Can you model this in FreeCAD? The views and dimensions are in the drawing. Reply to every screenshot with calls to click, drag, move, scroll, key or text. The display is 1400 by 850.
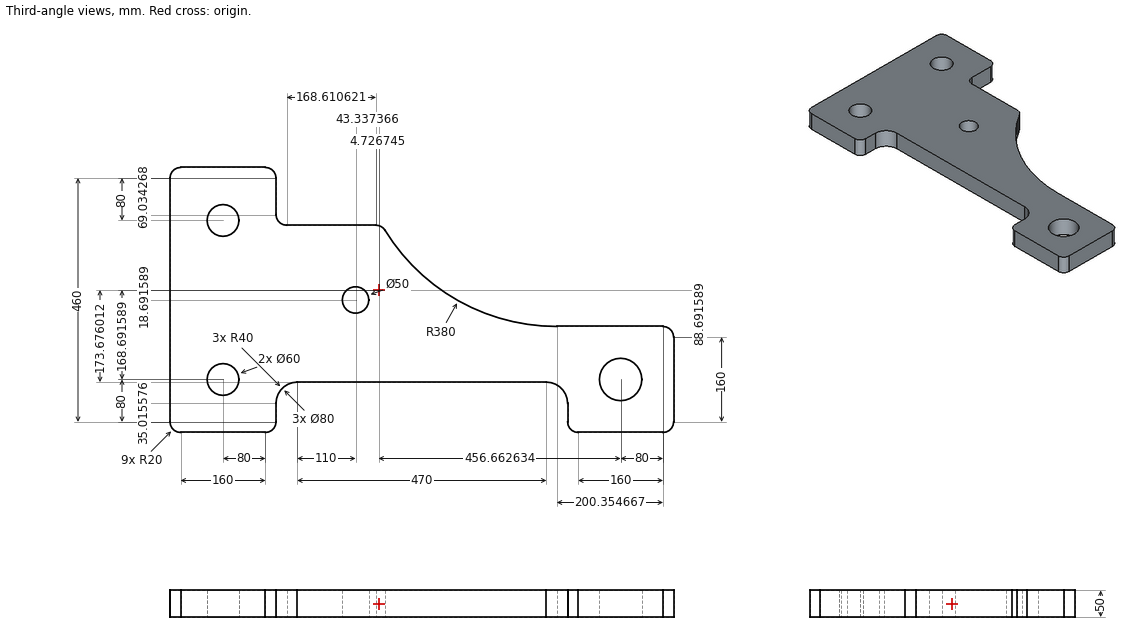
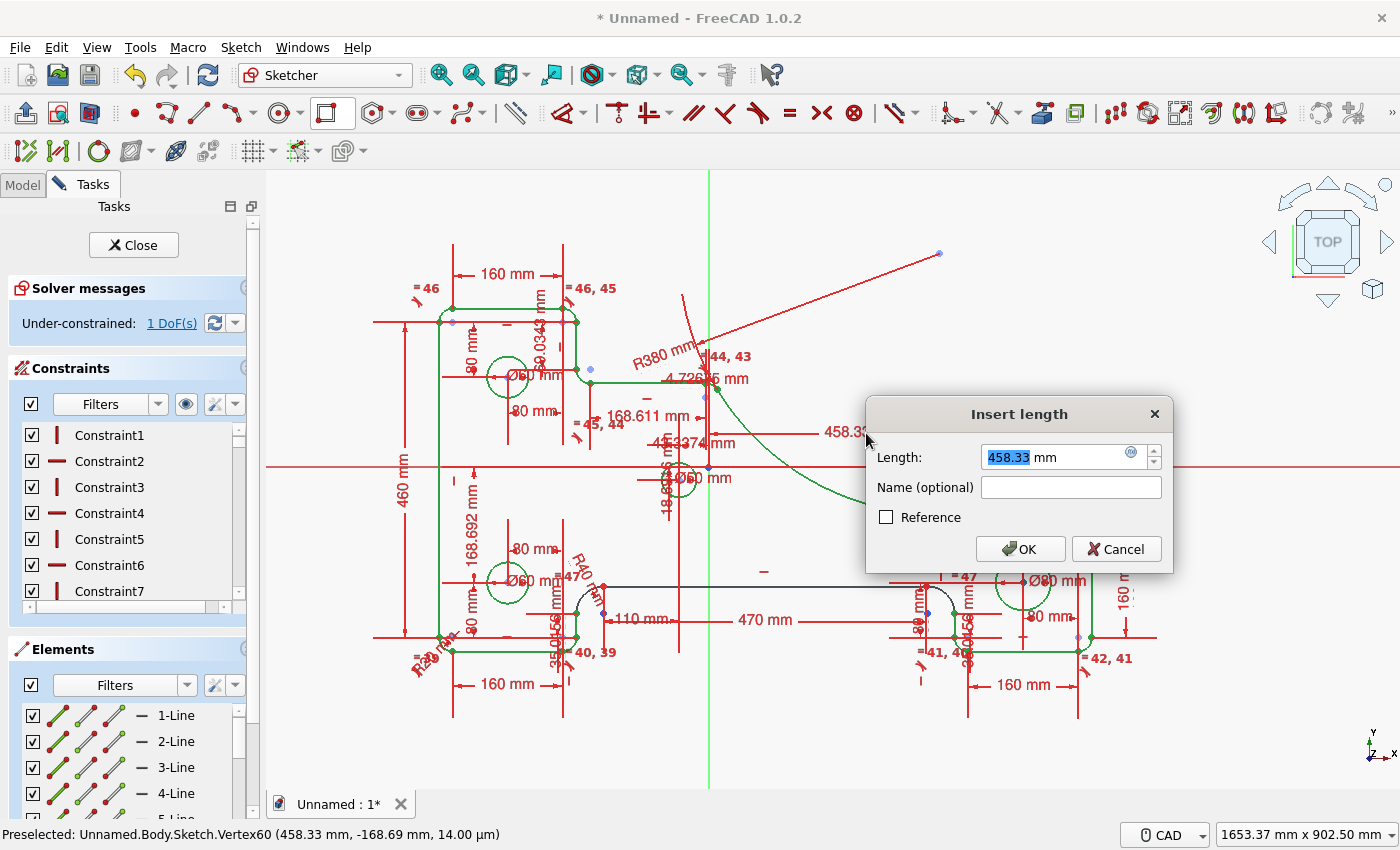
text(456.662634)
key(Return)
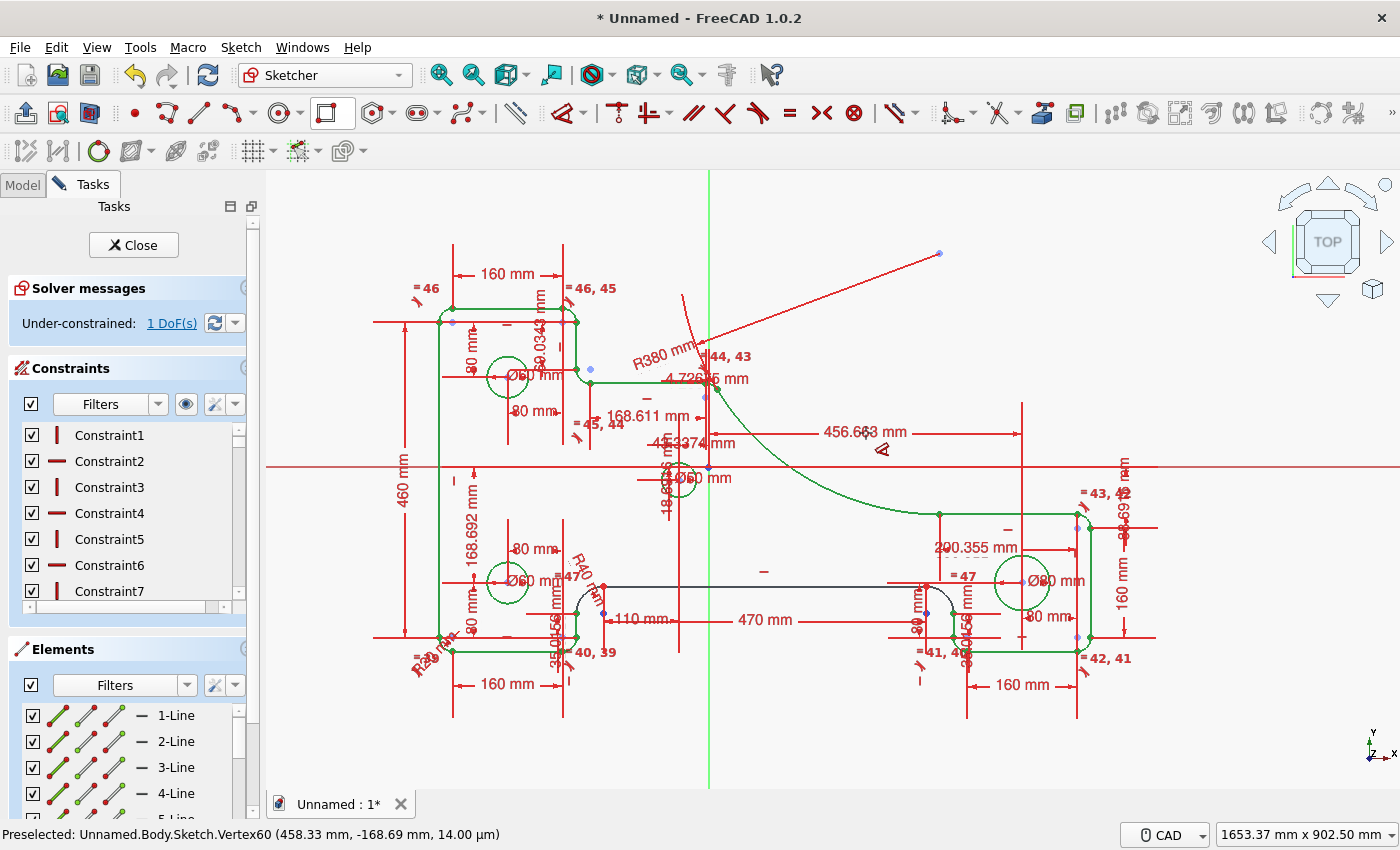
click(604, 587)
click(570, 527)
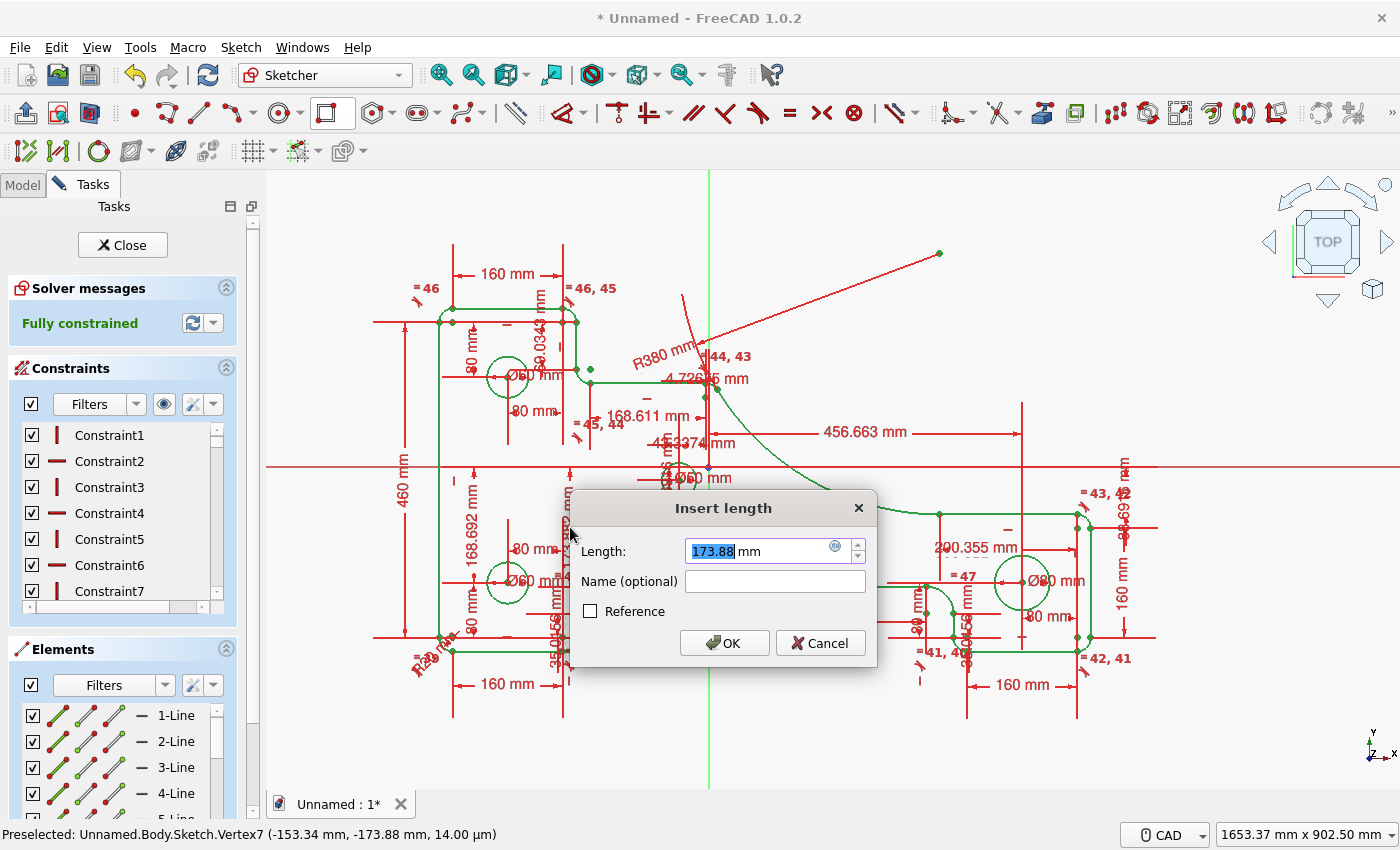
text(173.676012)
key(Return)
key(Escape)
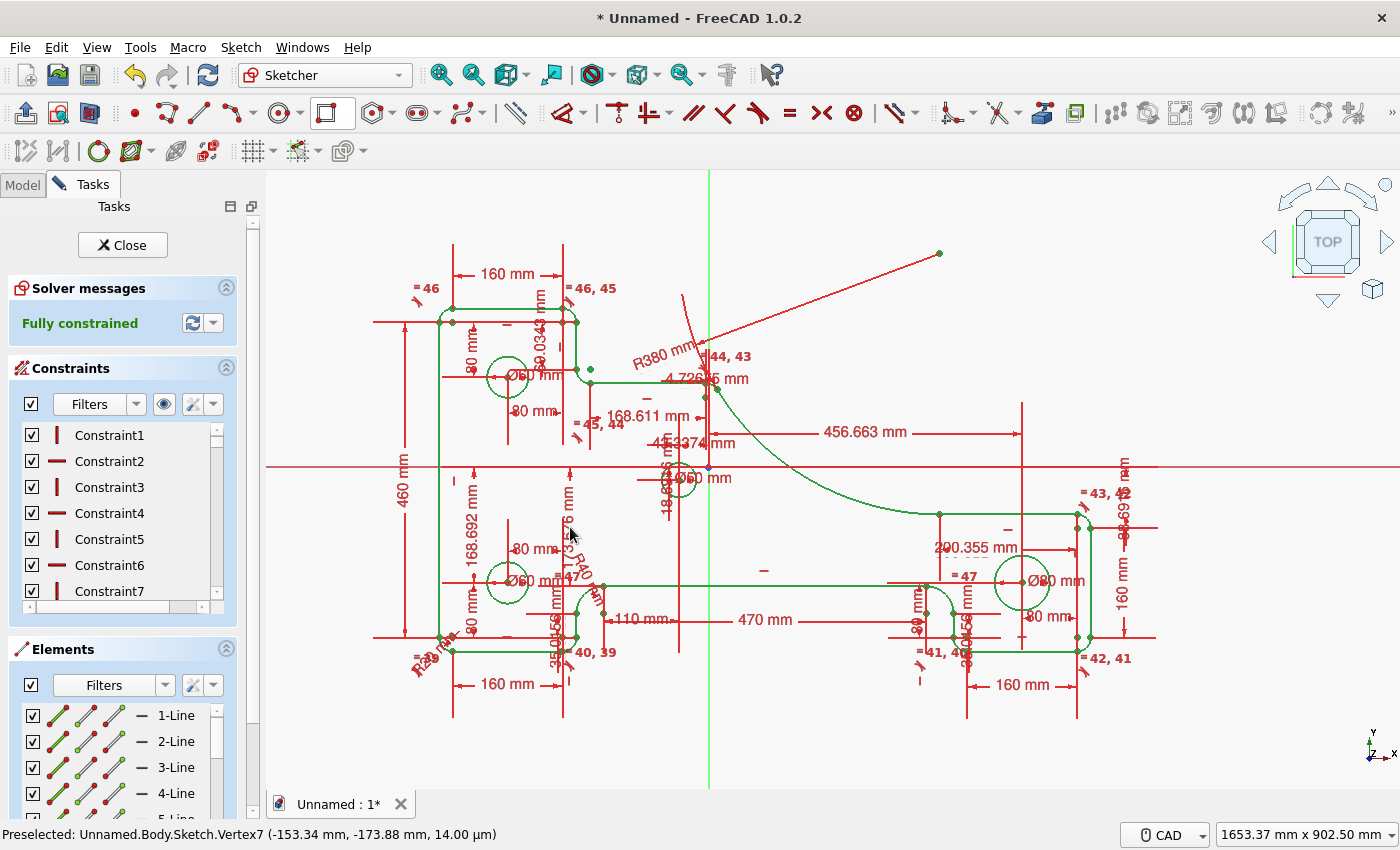
click(123, 245)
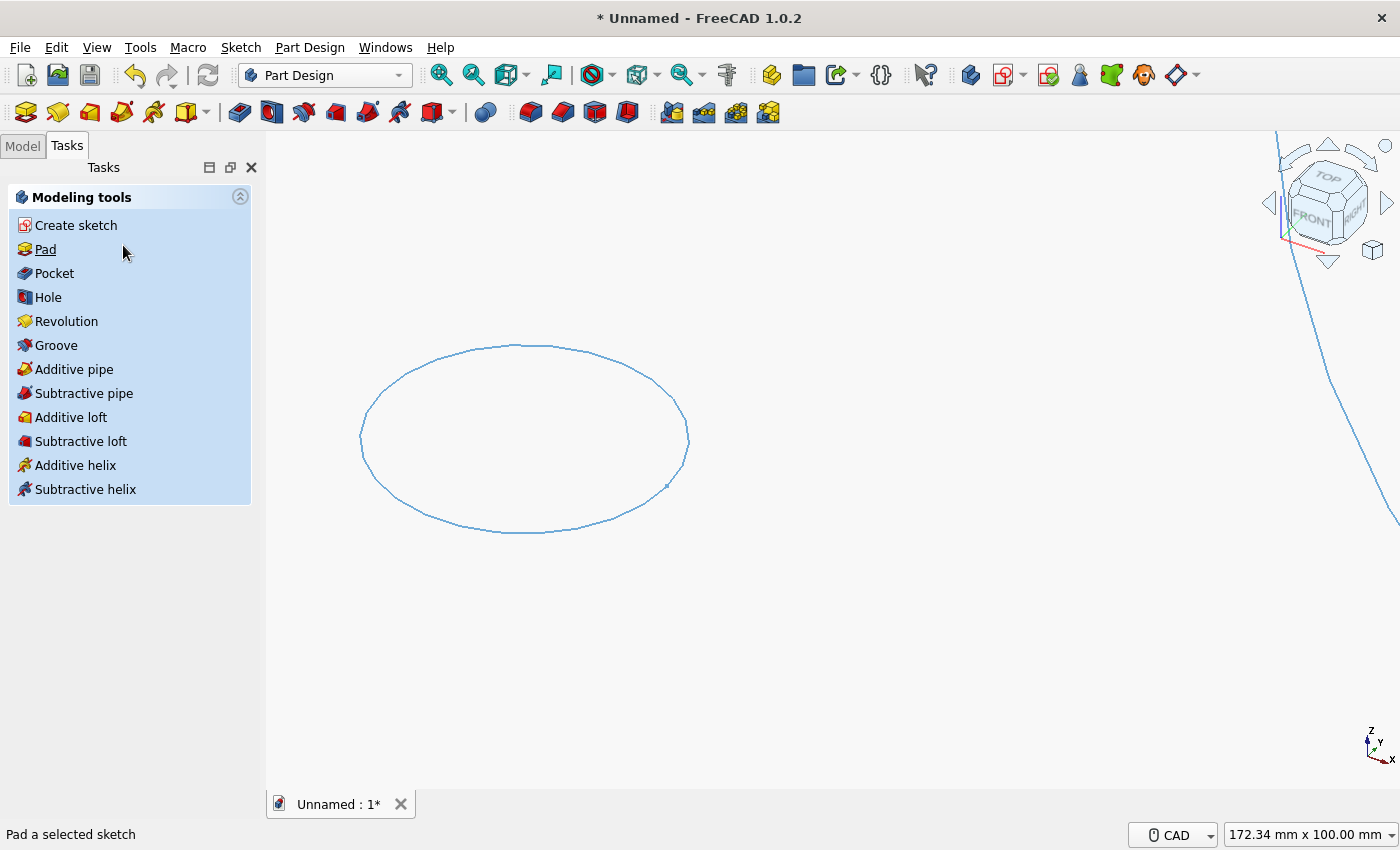
click(26, 112)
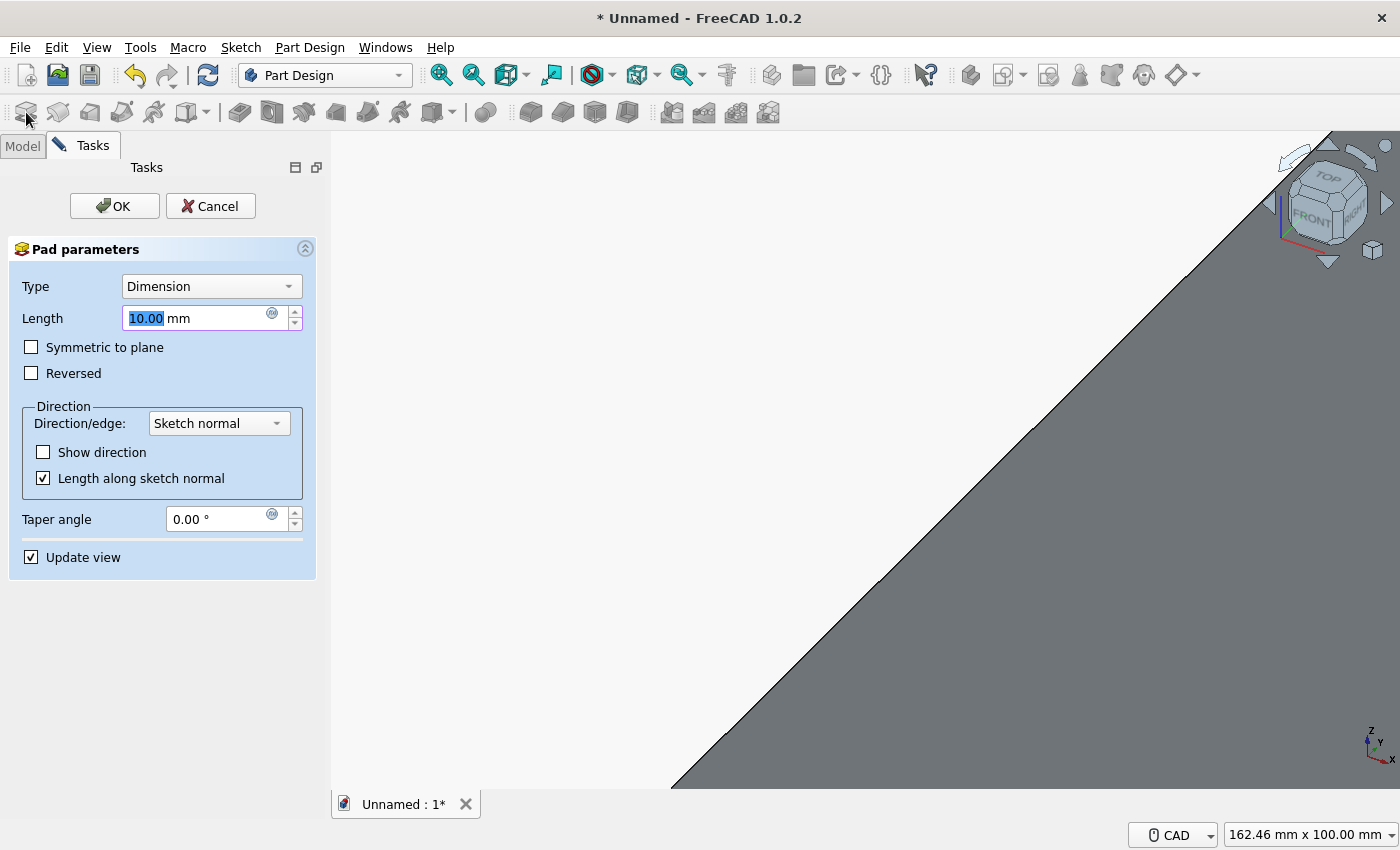
text(50)
key(Tab)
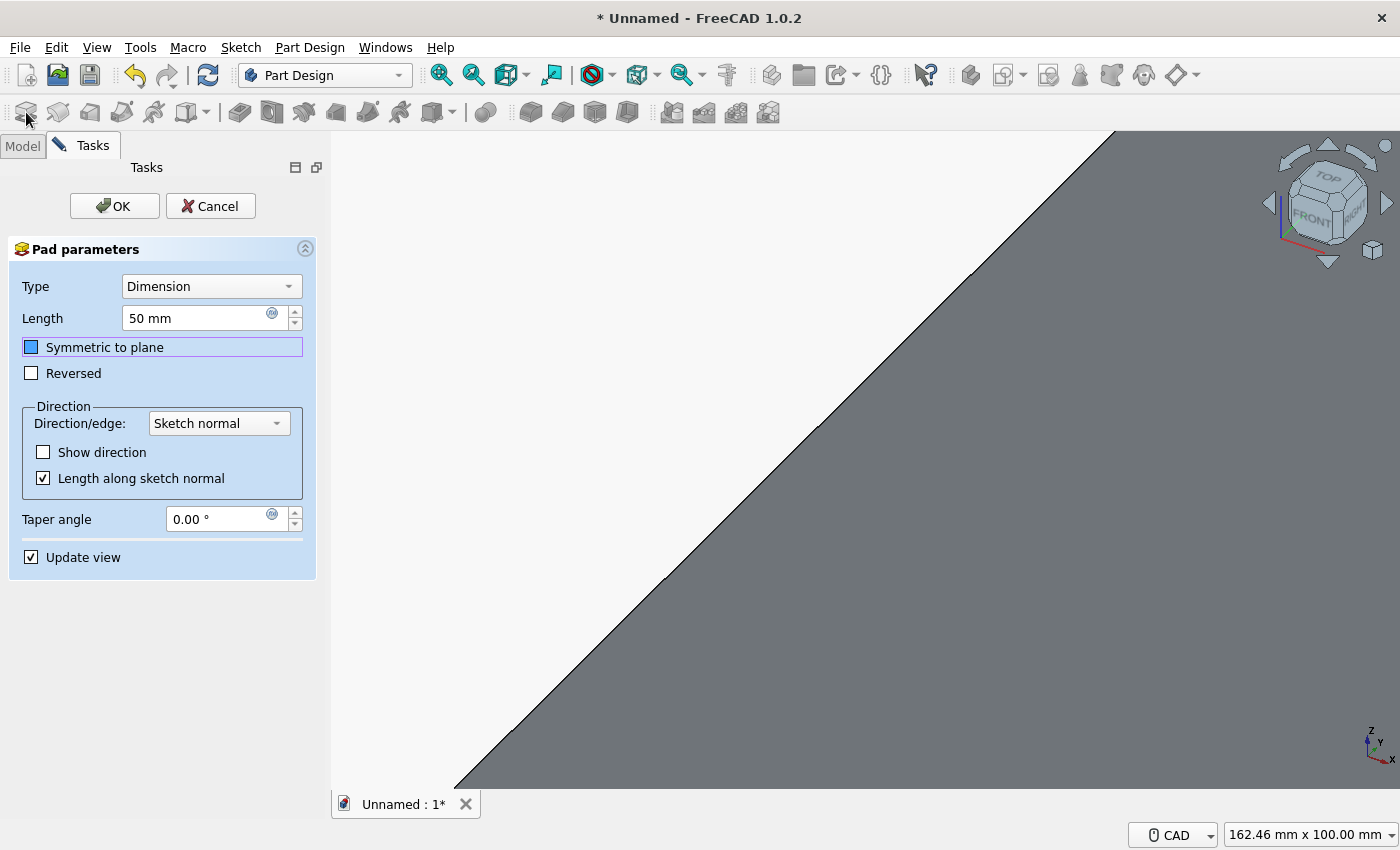
click(30, 347)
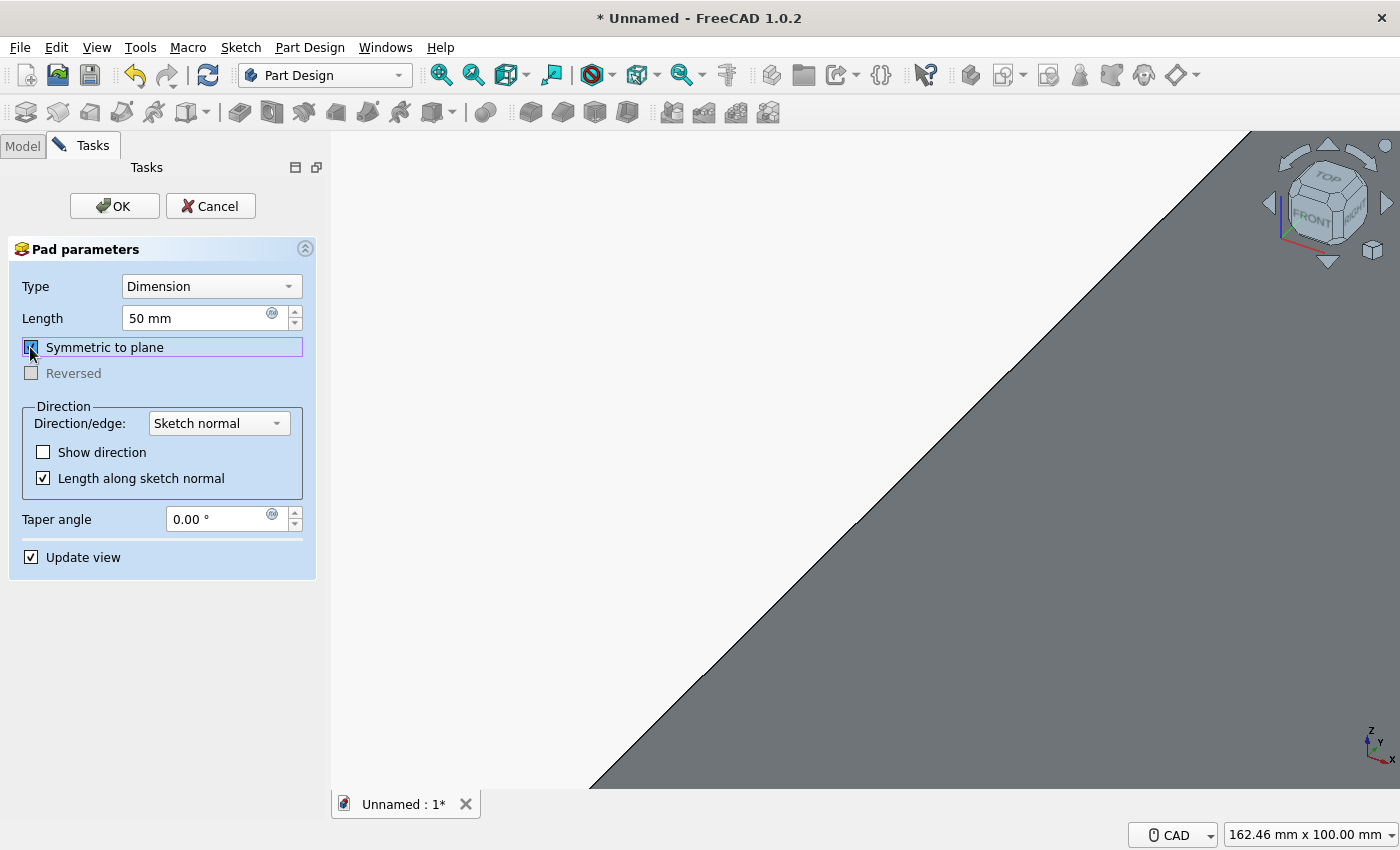
click(115, 206)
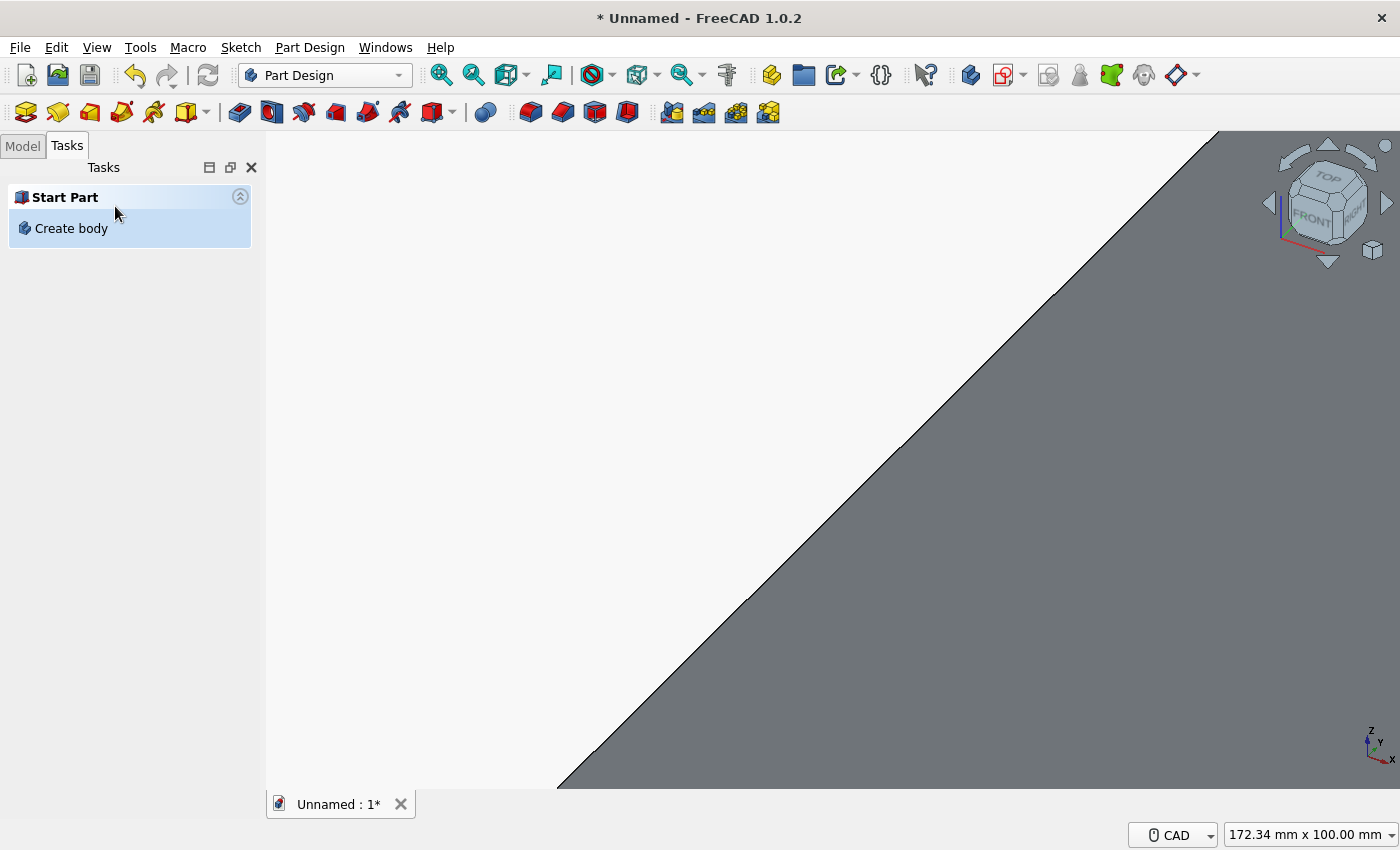
key(0)